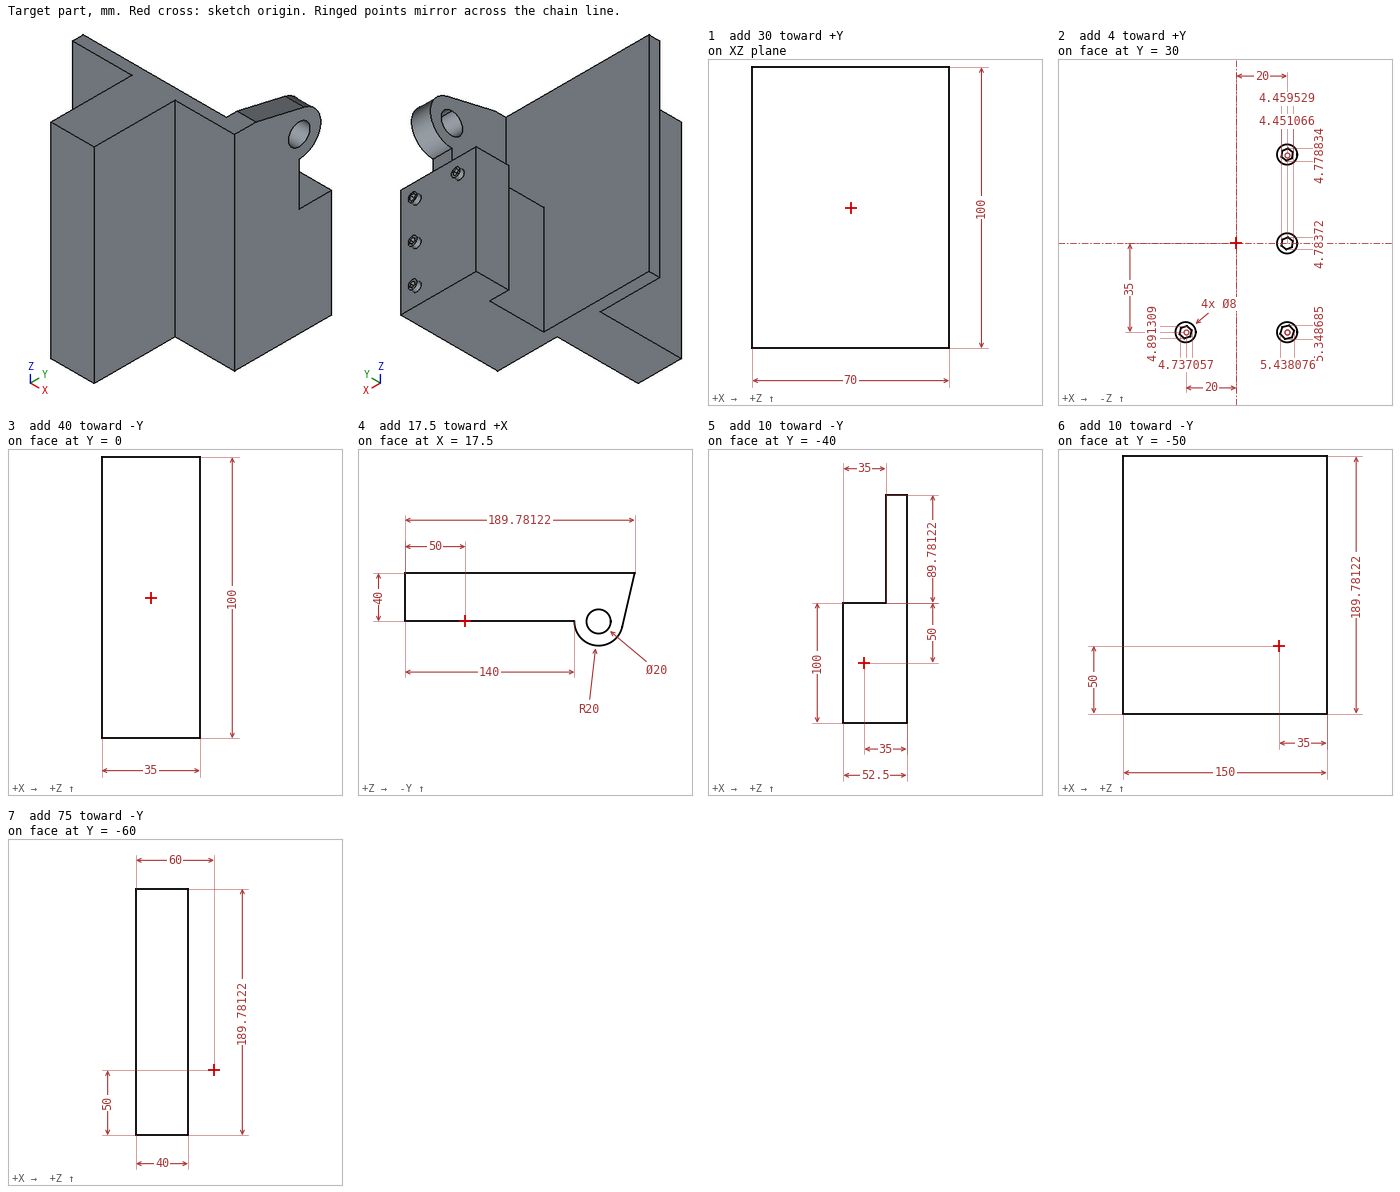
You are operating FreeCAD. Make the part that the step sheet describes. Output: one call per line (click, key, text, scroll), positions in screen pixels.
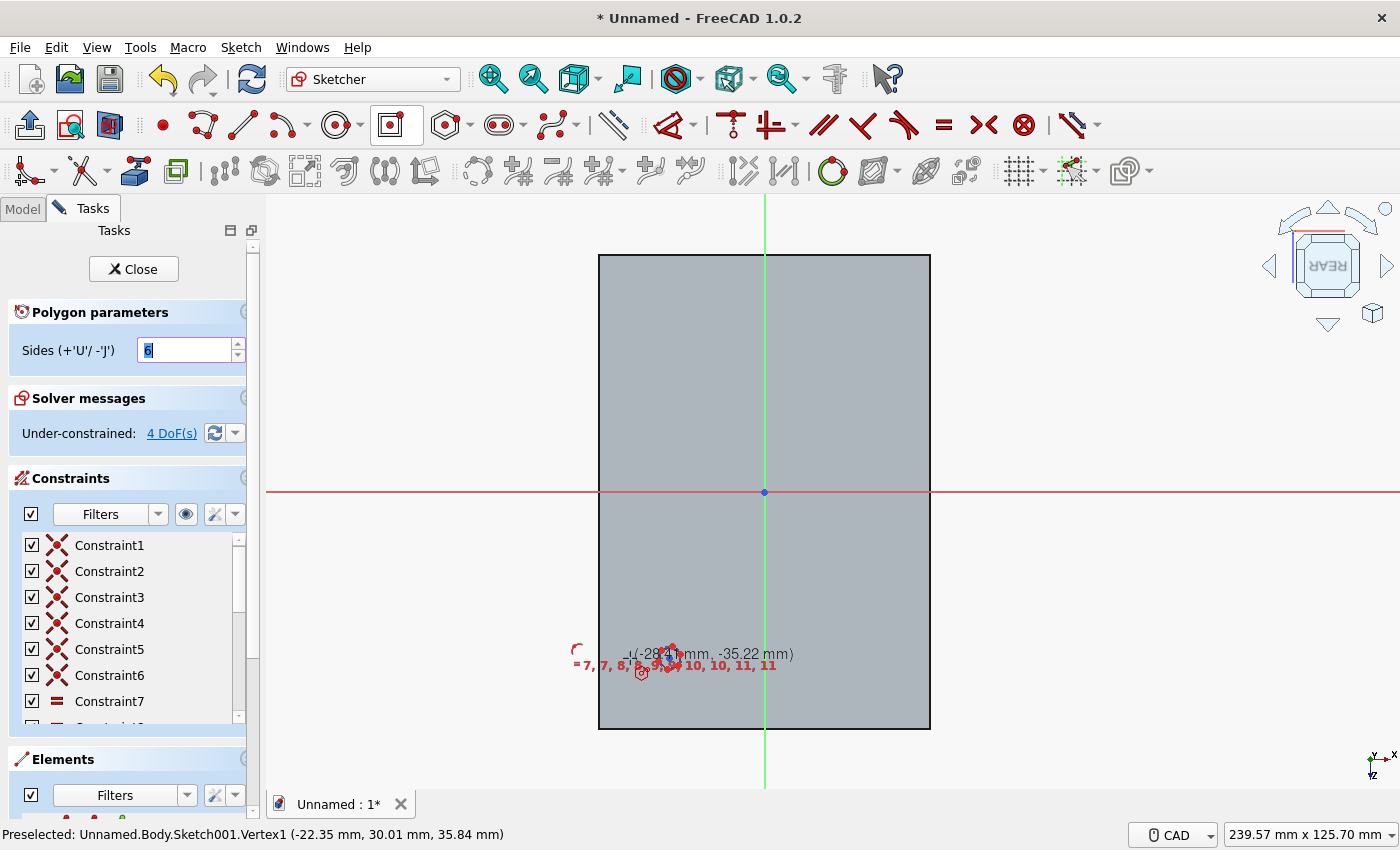
scroll(859, 658, up, 5)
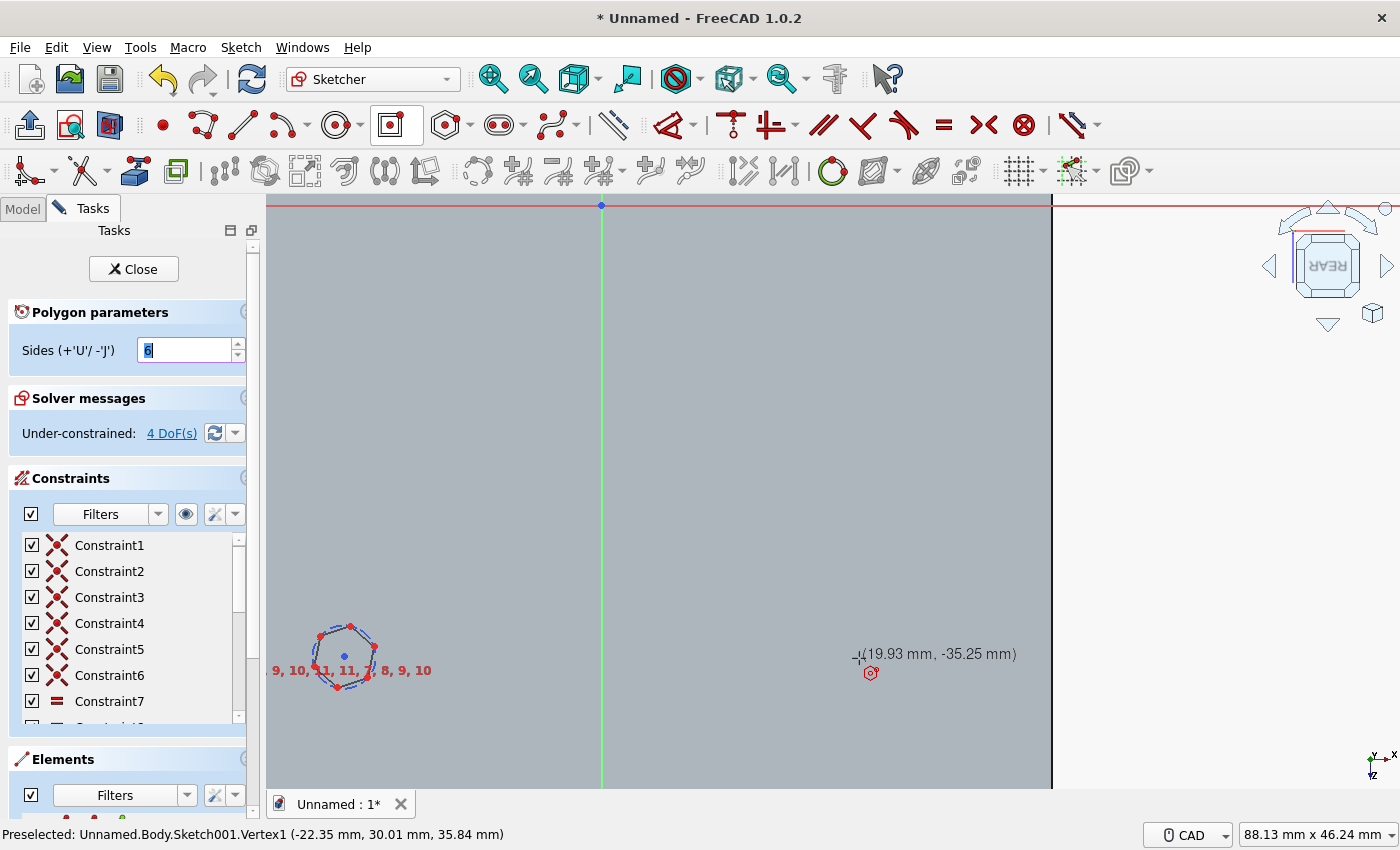
click(859, 656)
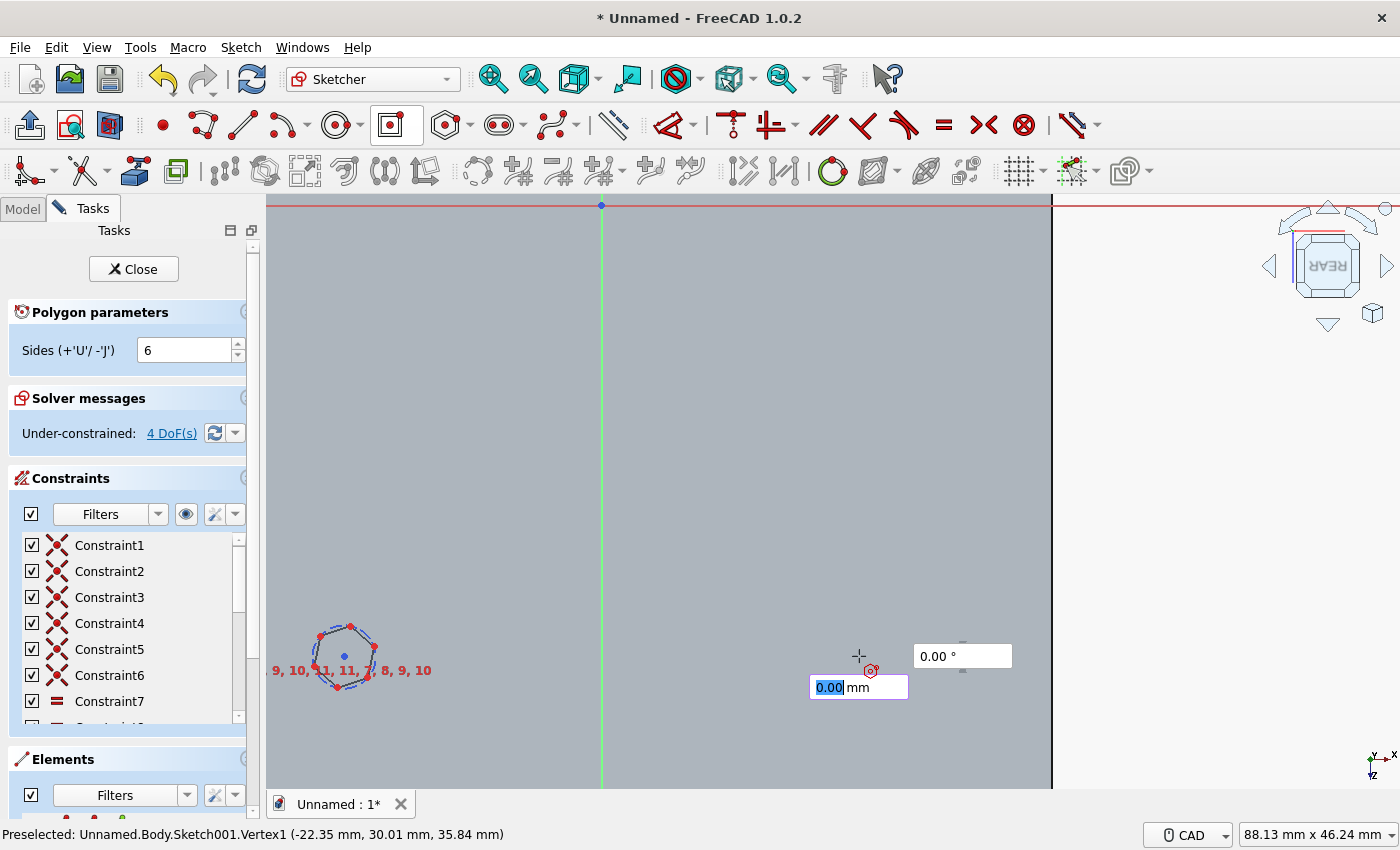
click(894, 648)
right_click(894, 648)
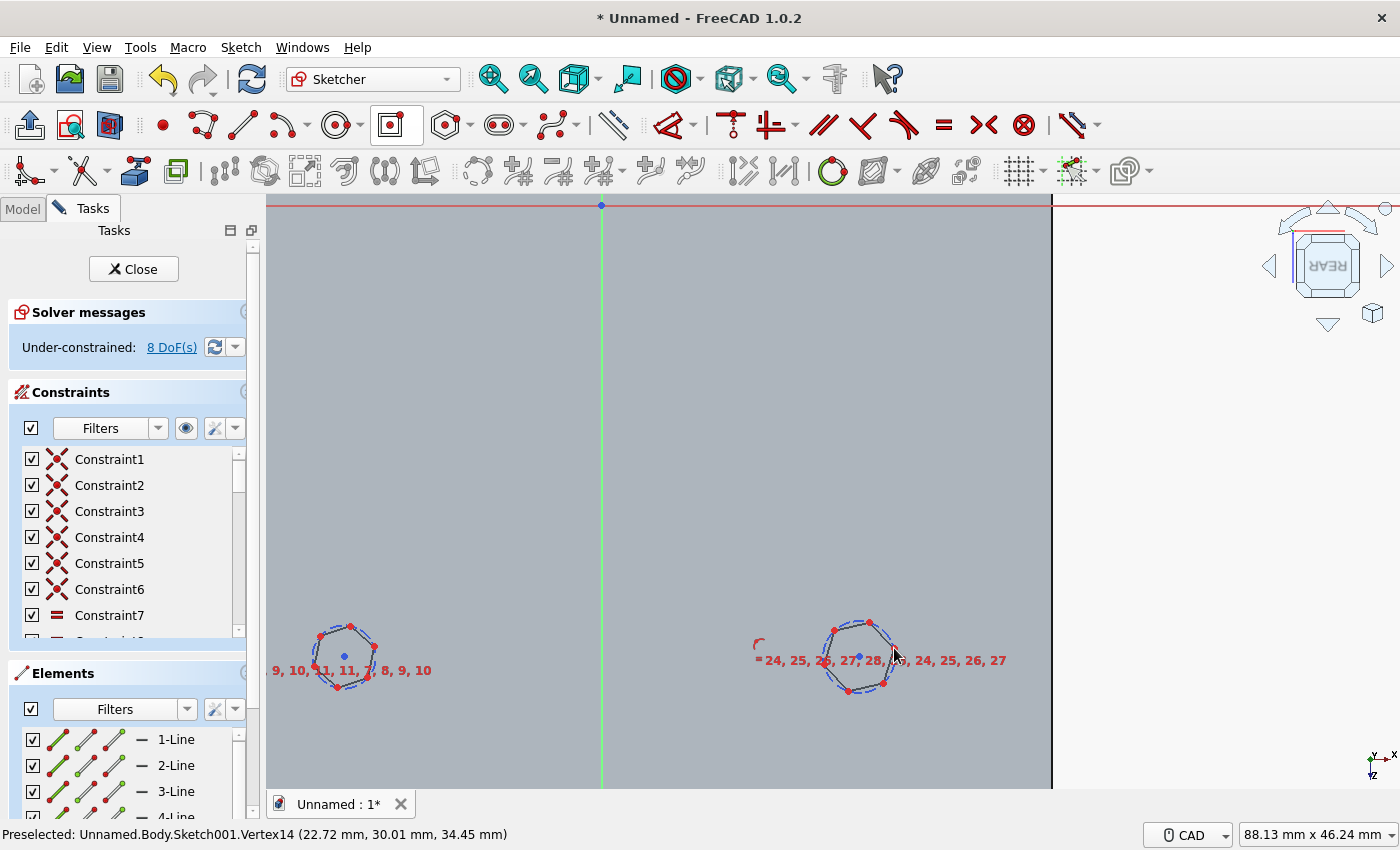
click(446, 126)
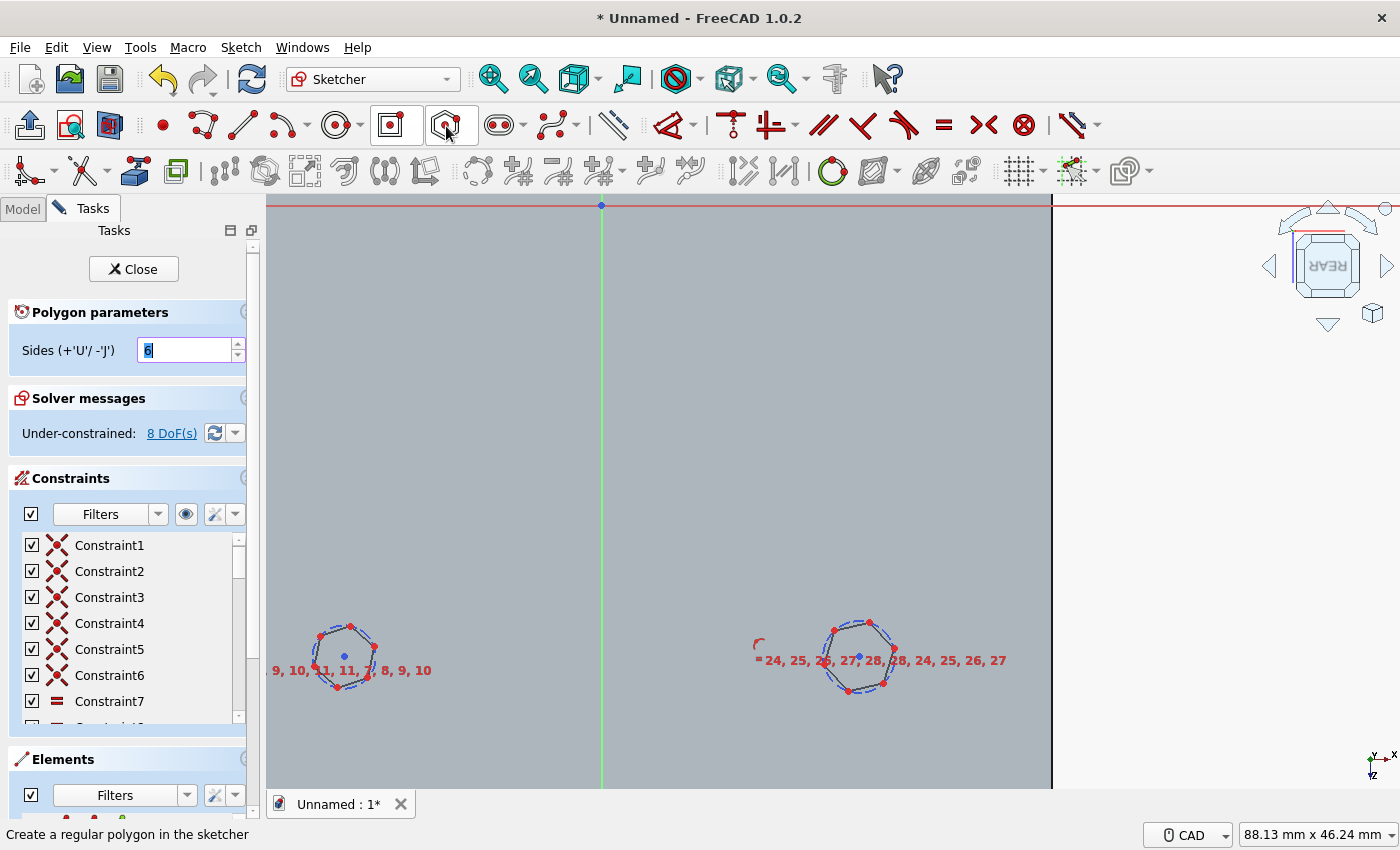
scroll(859, 658, down, 5)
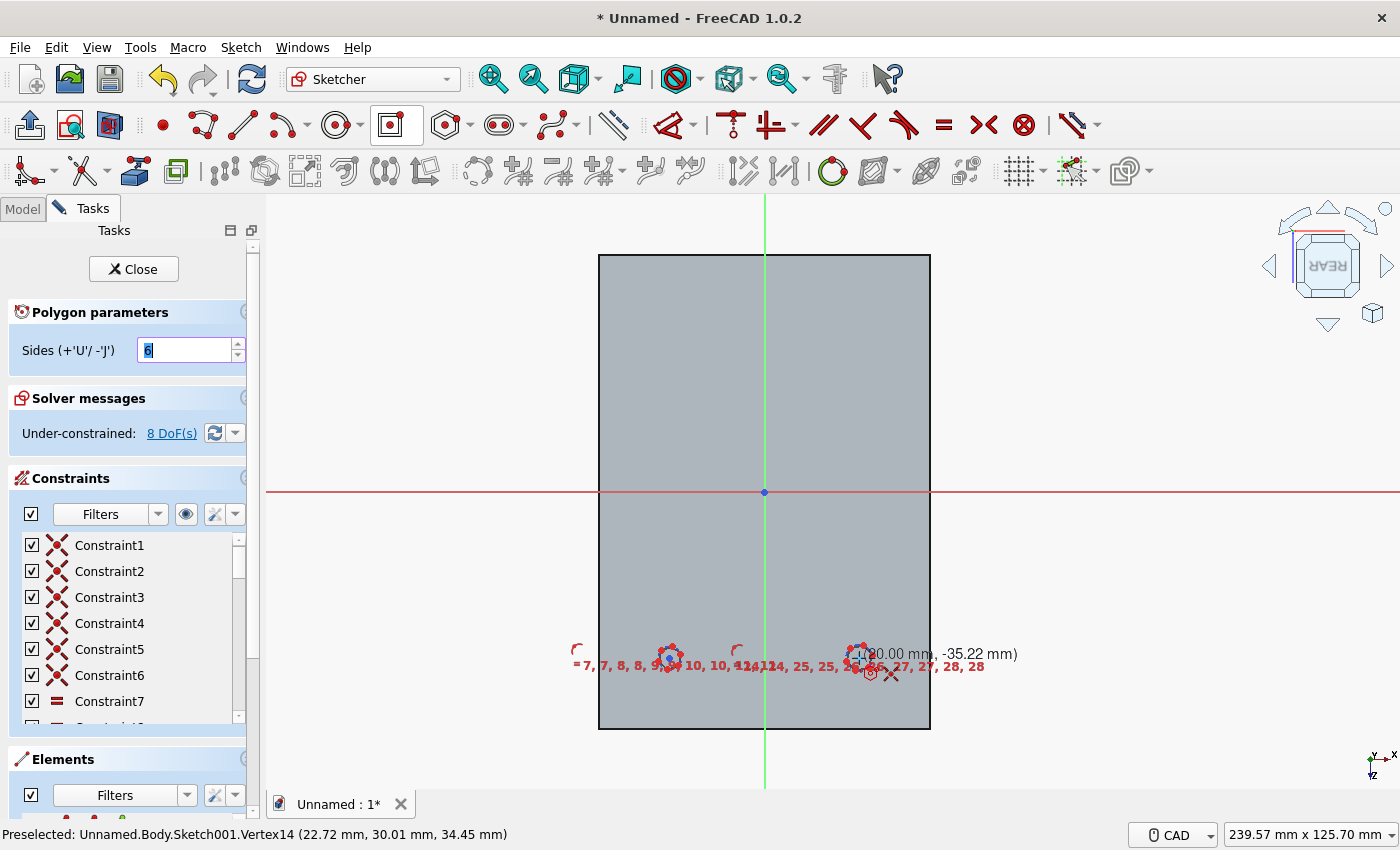
scroll(859, 492, up, 6)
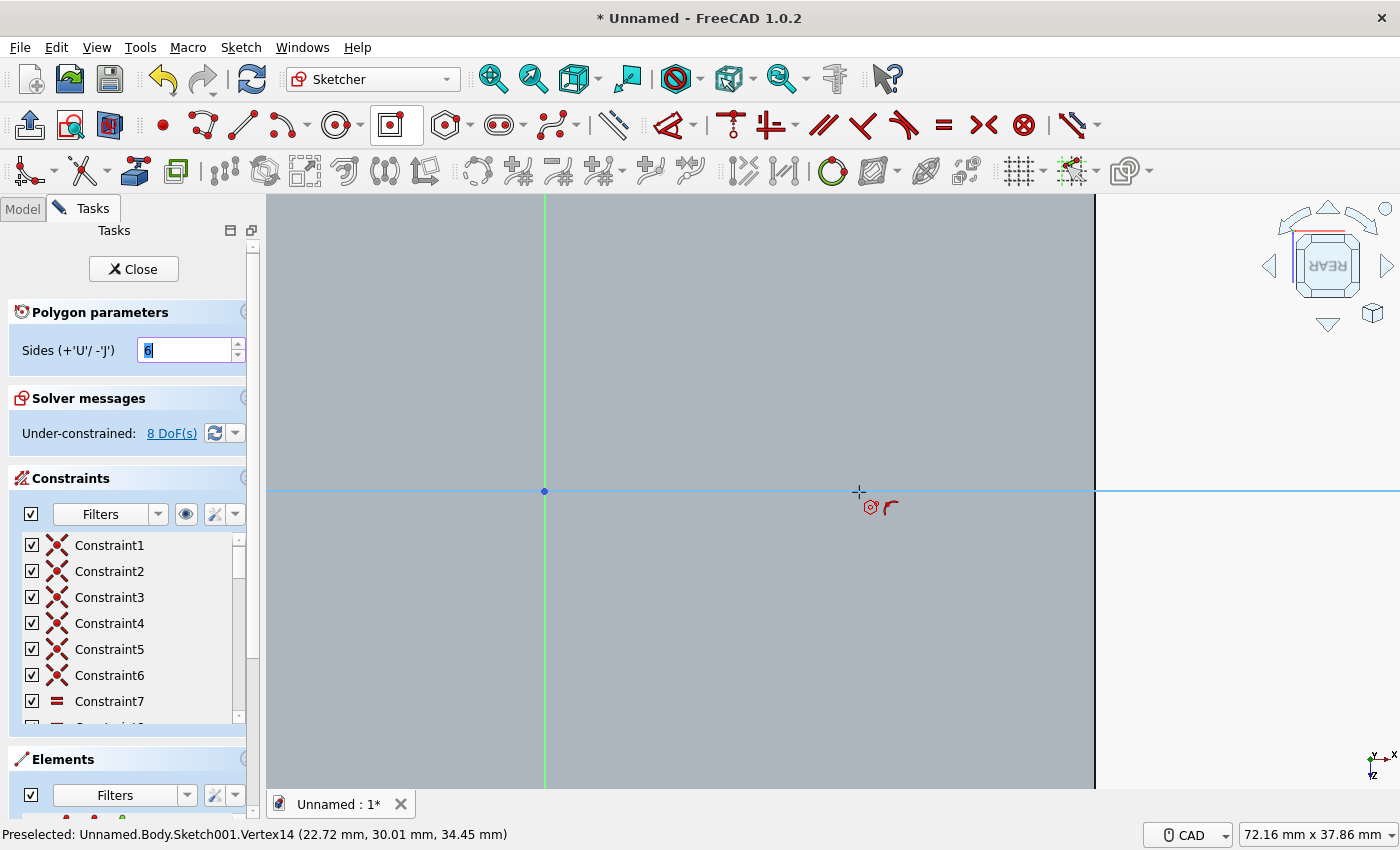
click(859, 491)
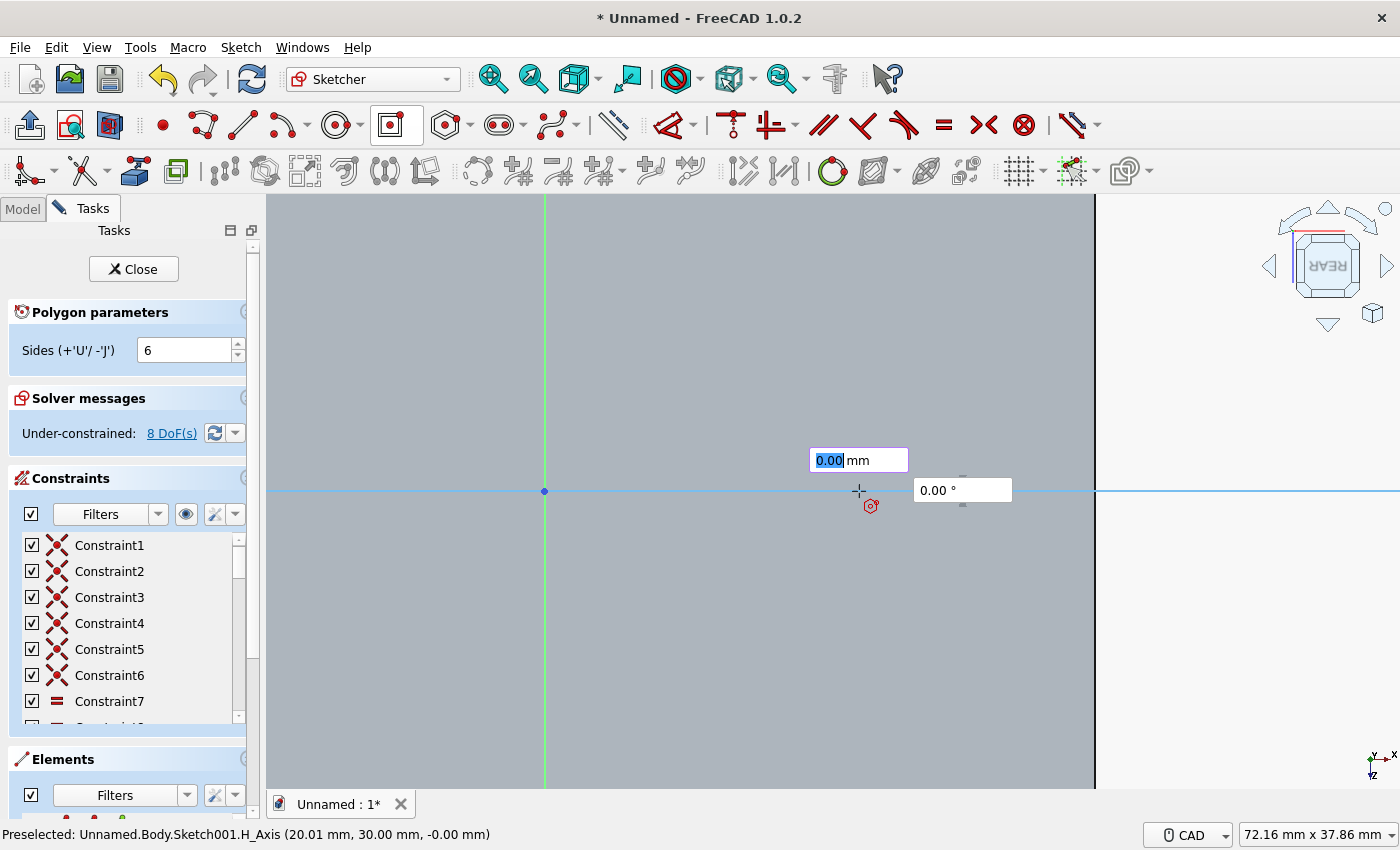
click(854, 529)
right_click(854, 529)